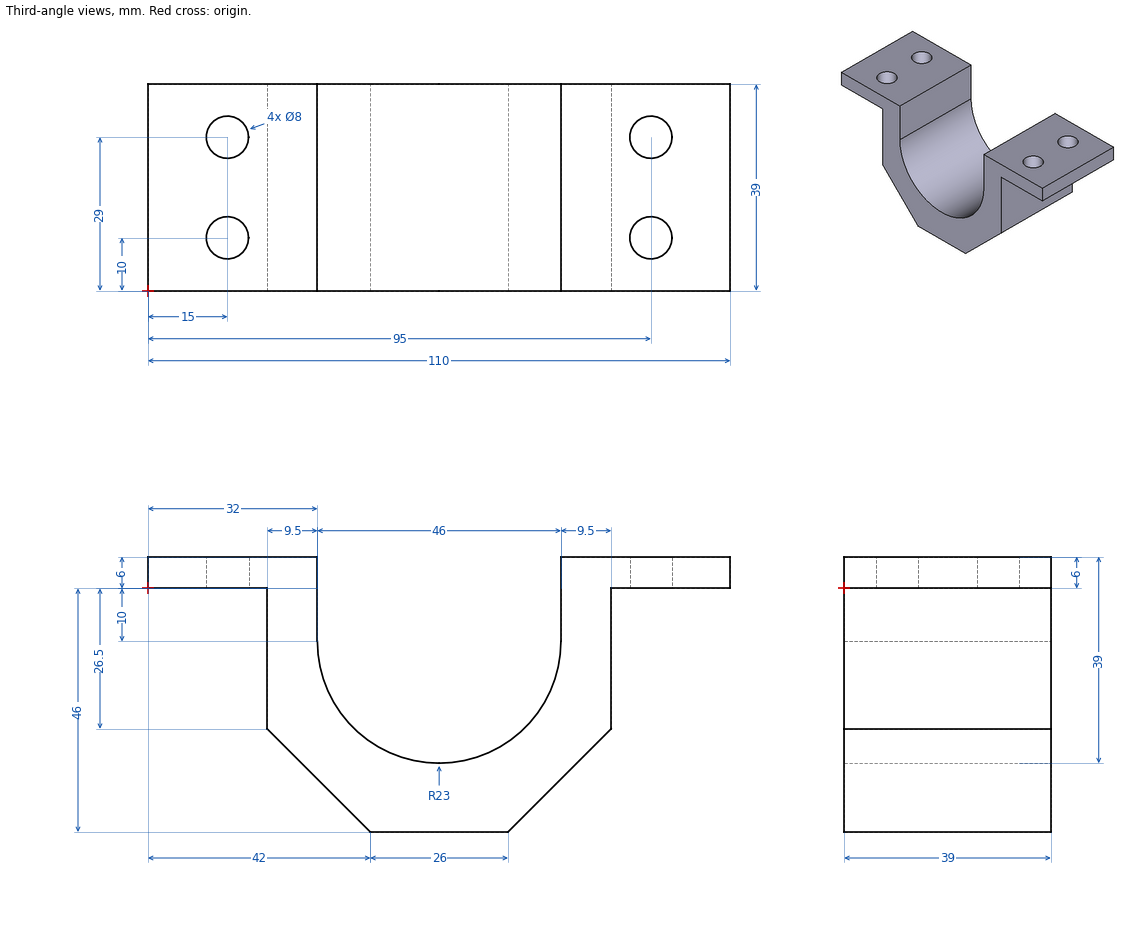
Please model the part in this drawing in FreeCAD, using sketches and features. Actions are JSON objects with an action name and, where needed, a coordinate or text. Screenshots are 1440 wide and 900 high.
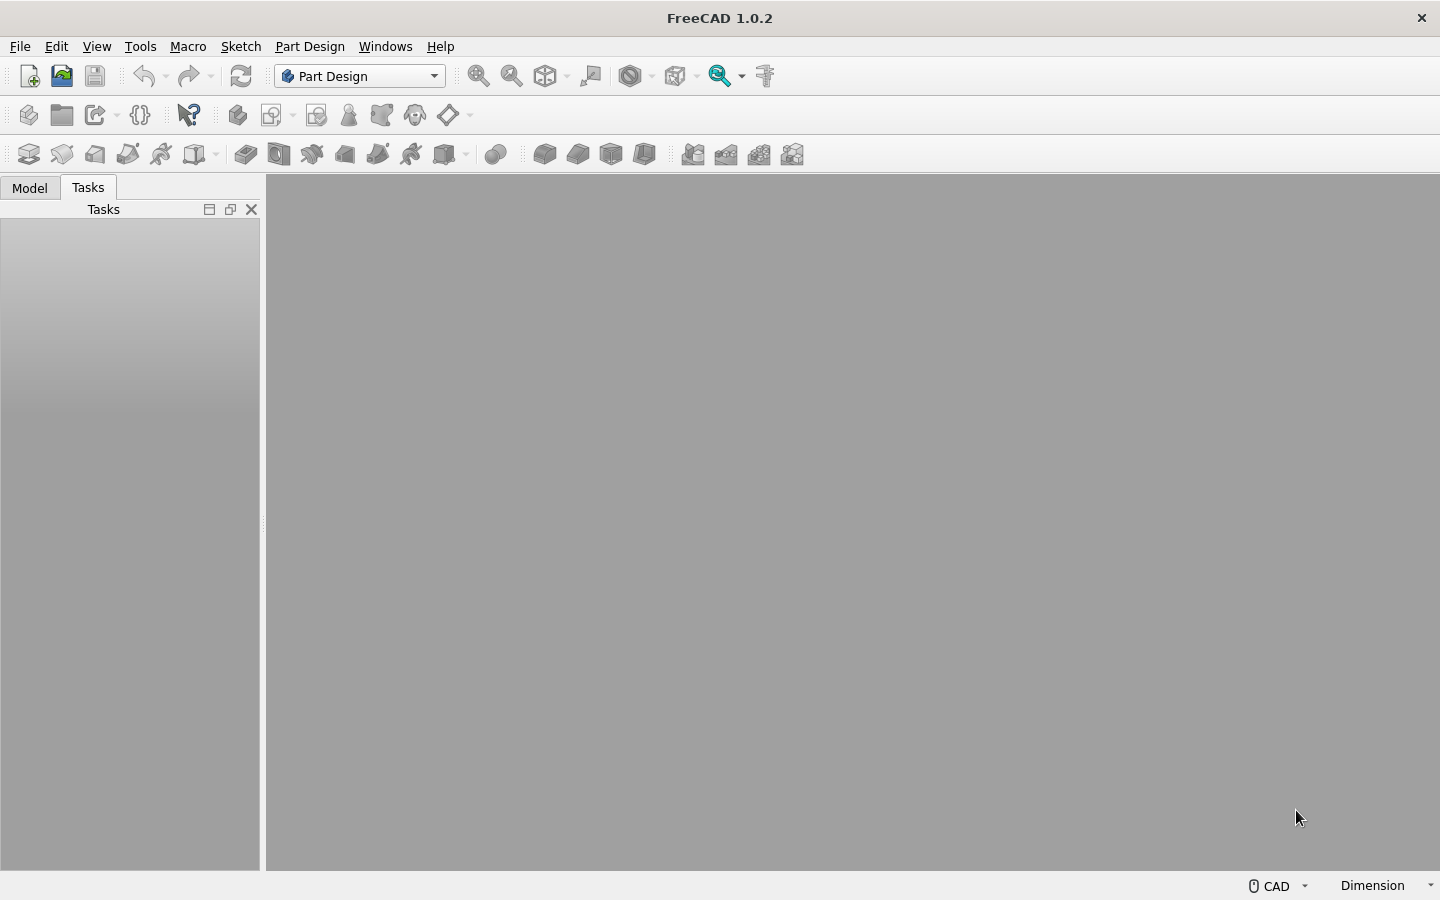
{"action": "key", "text": "ctrl+n"}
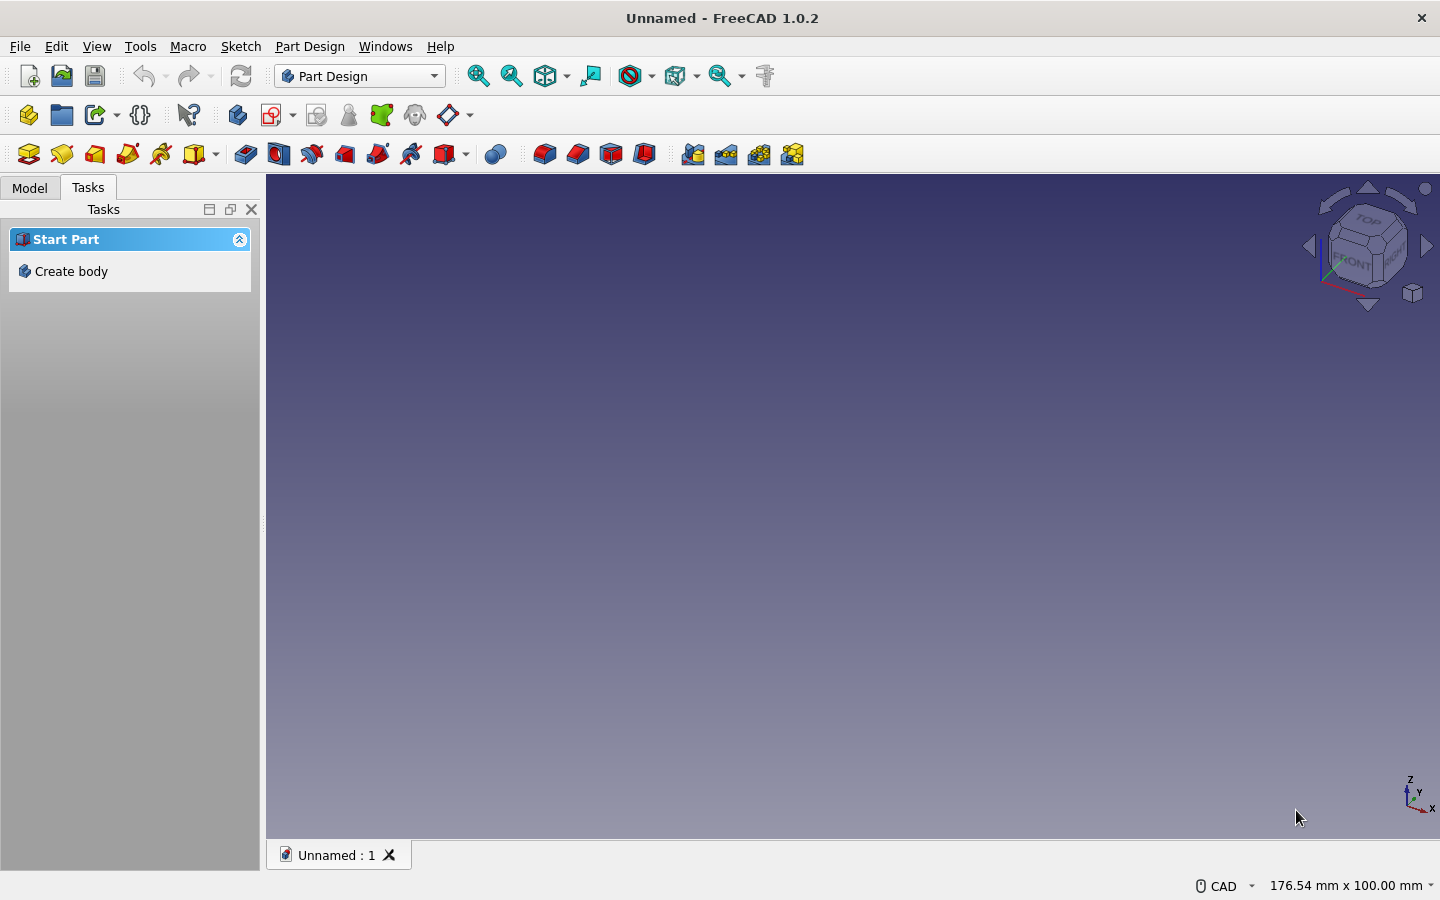
{"action": "left_click", "coordinate": [270, 116]}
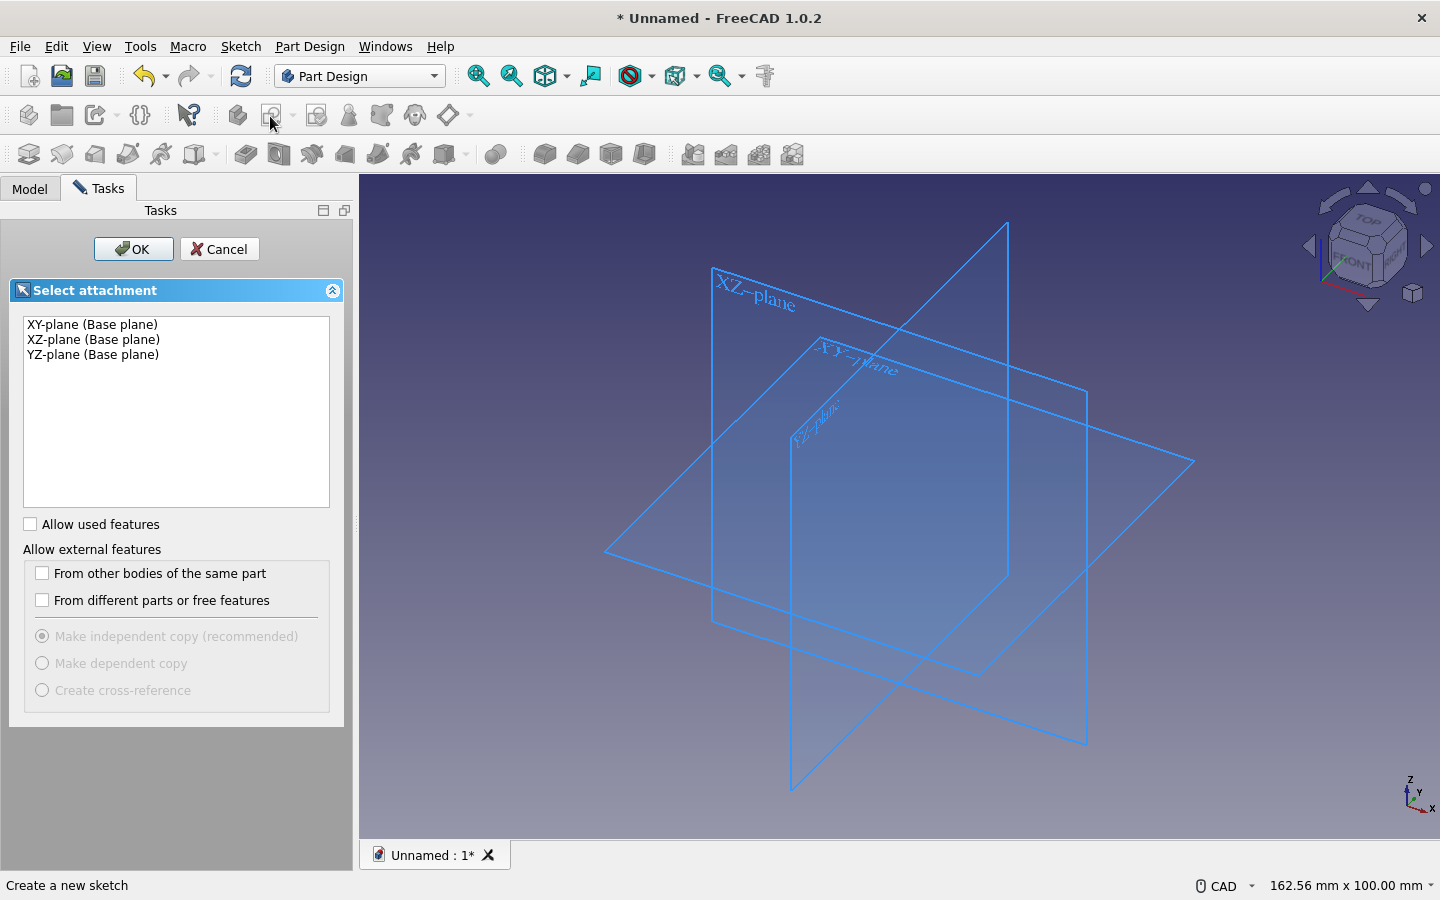
{"action": "left_click", "coordinate": [84, 324]}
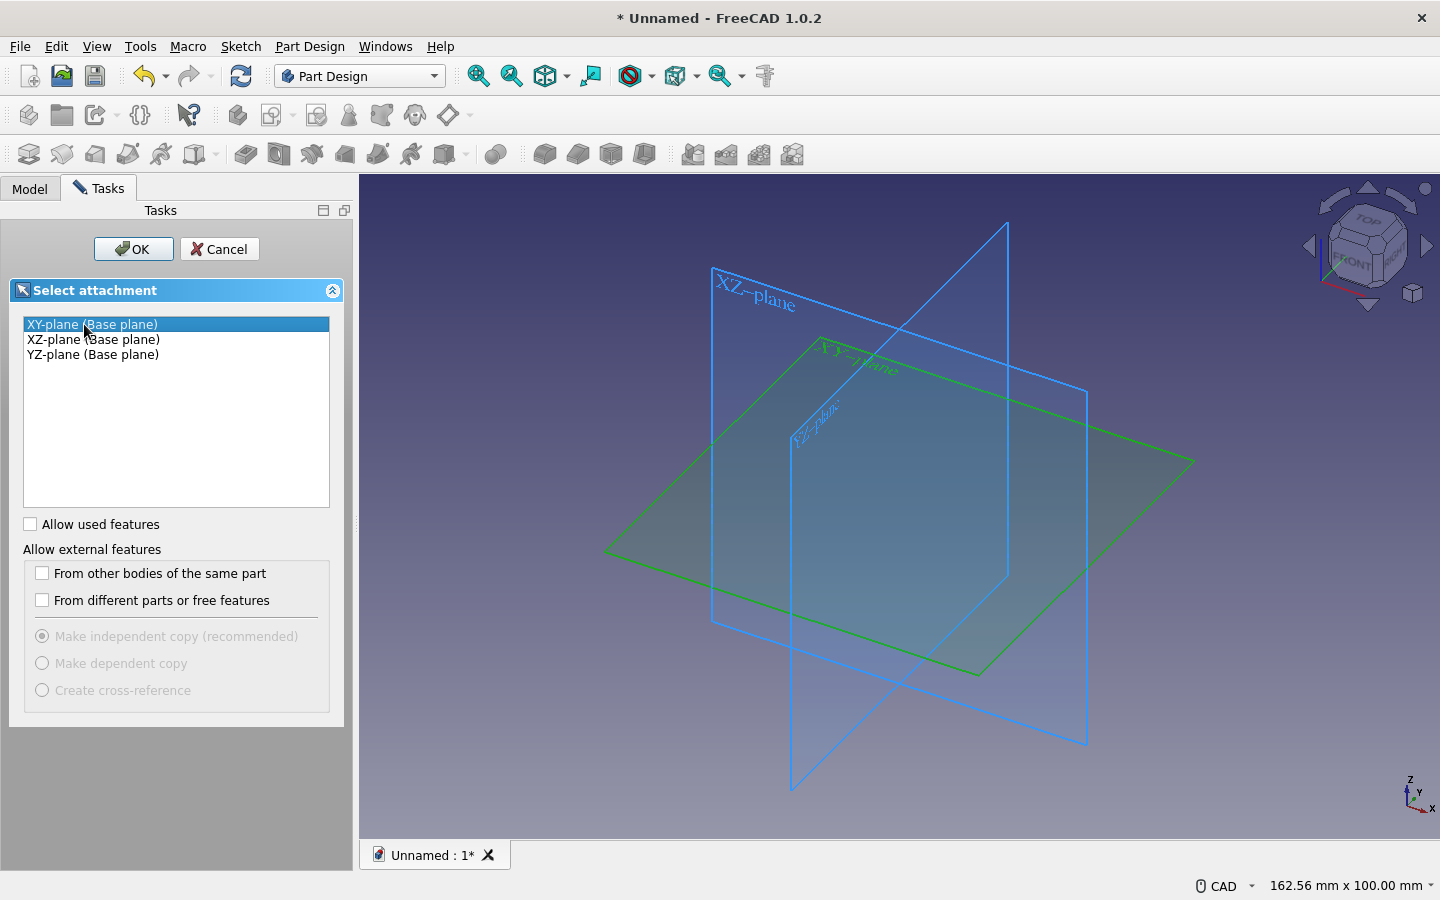
{"action": "left_click", "coordinate": [134, 249]}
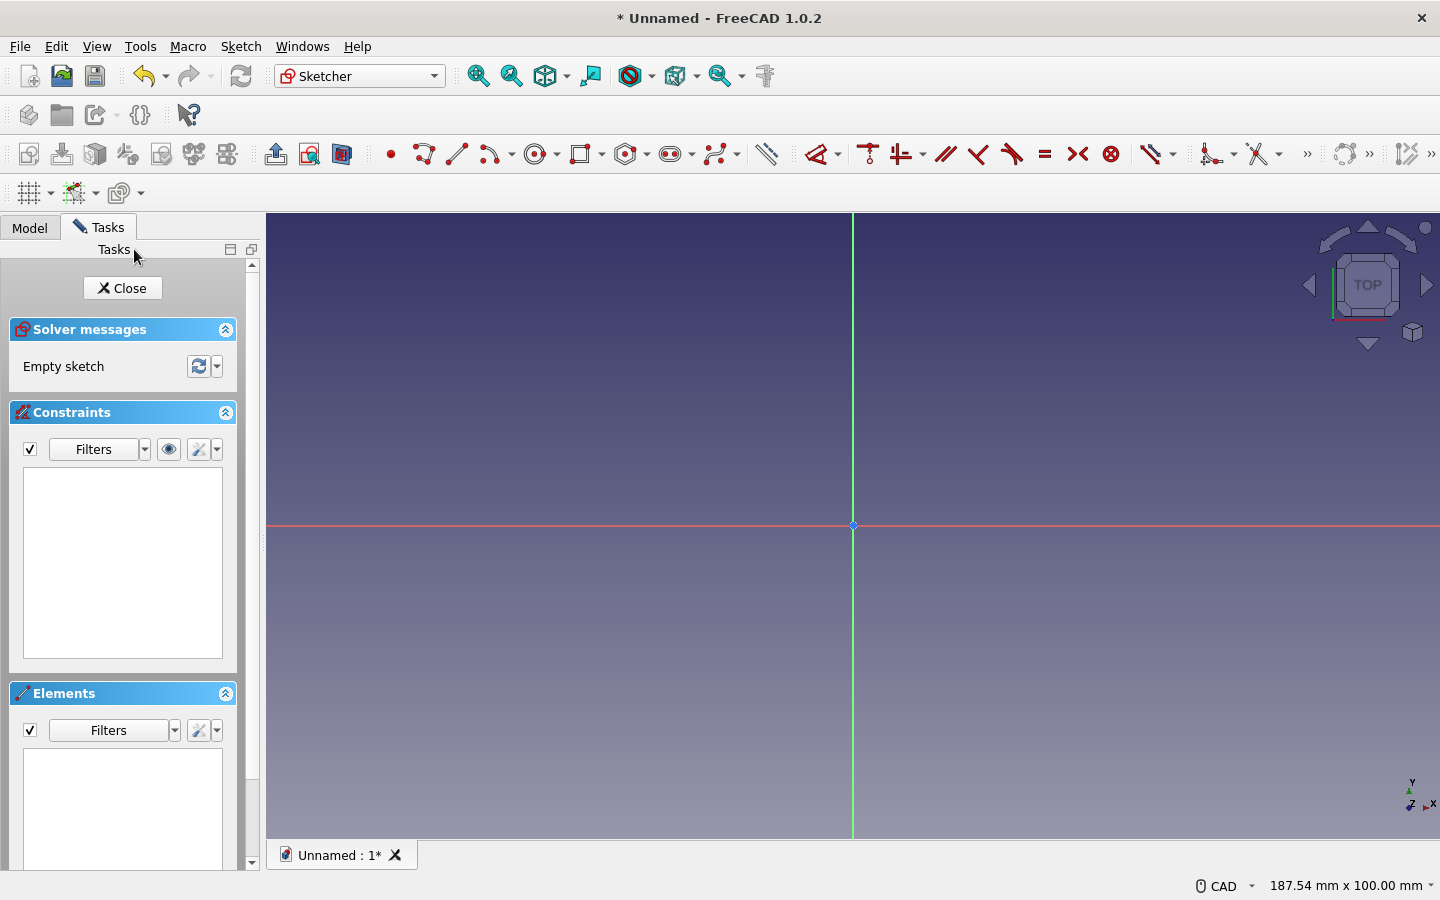
{"action": "scroll", "coordinate": [294, 774], "scroll_direction": "down", "scroll_amount": 2}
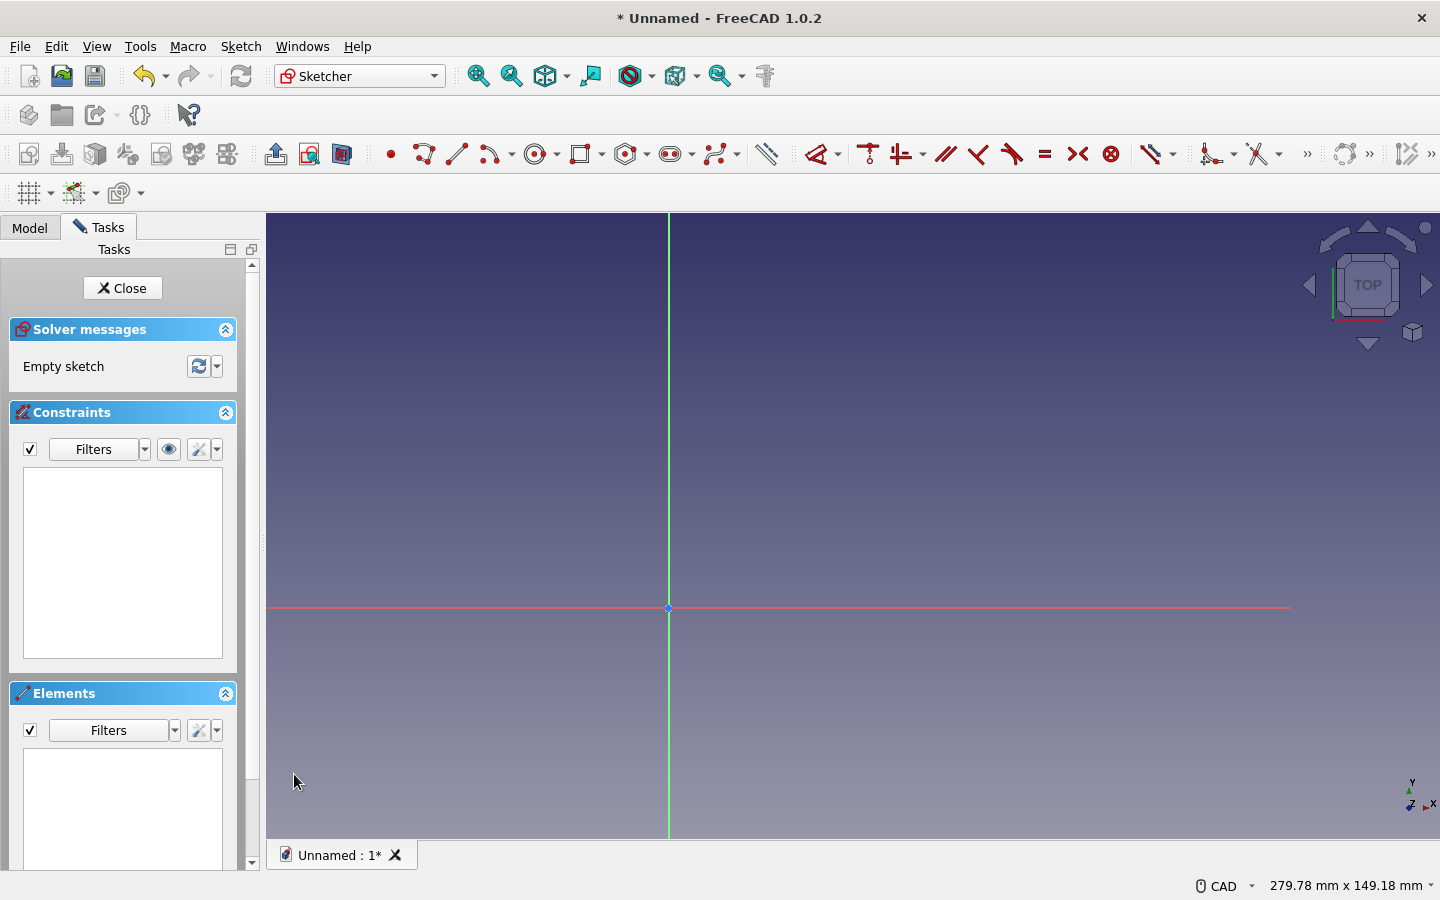
{"action": "scroll", "coordinate": [1133, 527], "scroll_direction": "up", "scroll_amount": 2}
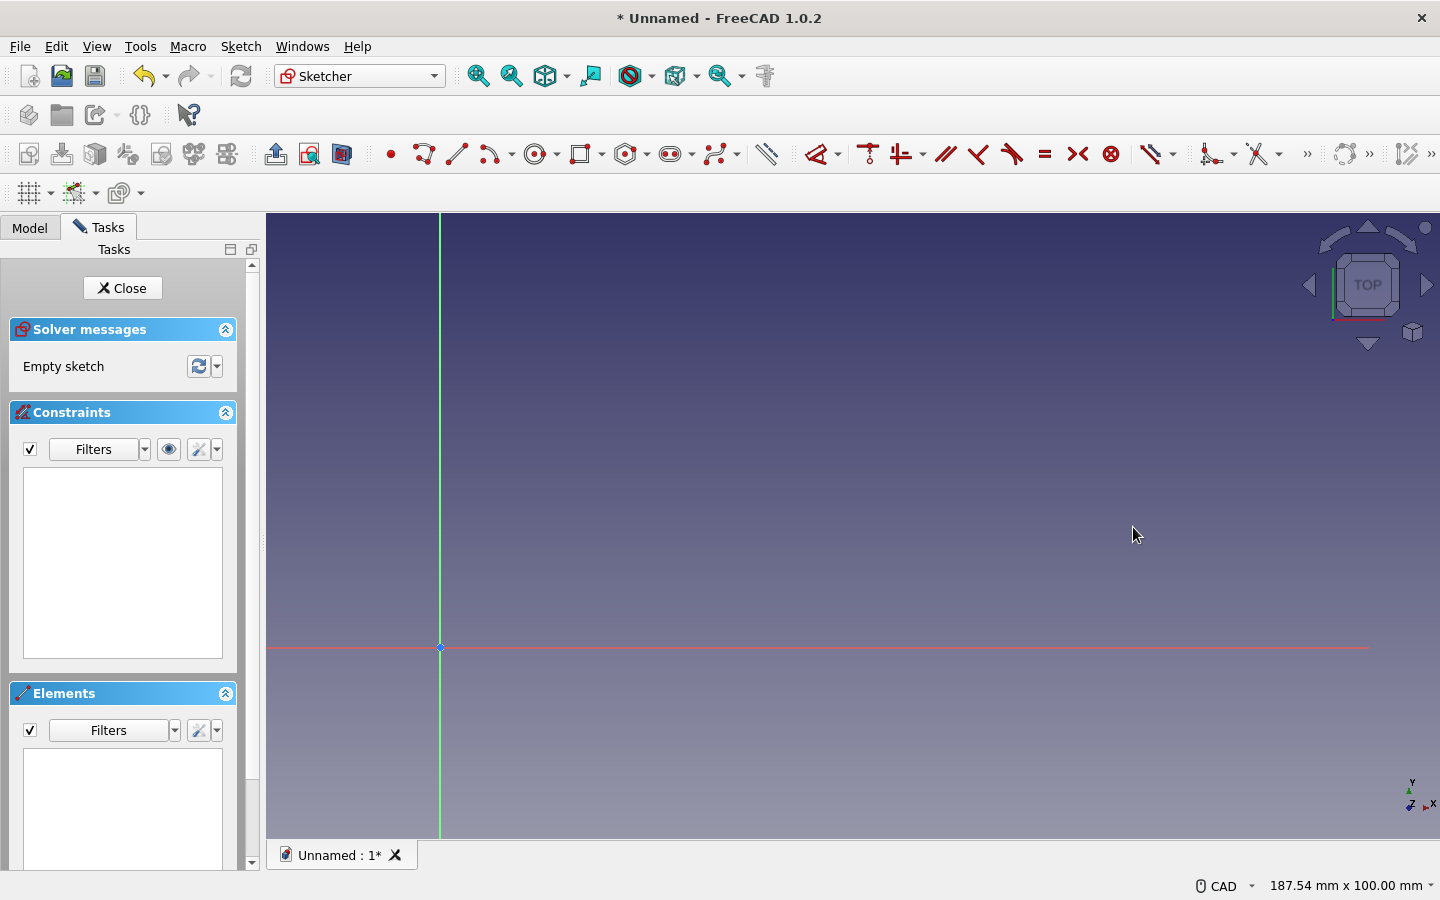
{"action": "key", "text": "g r"}